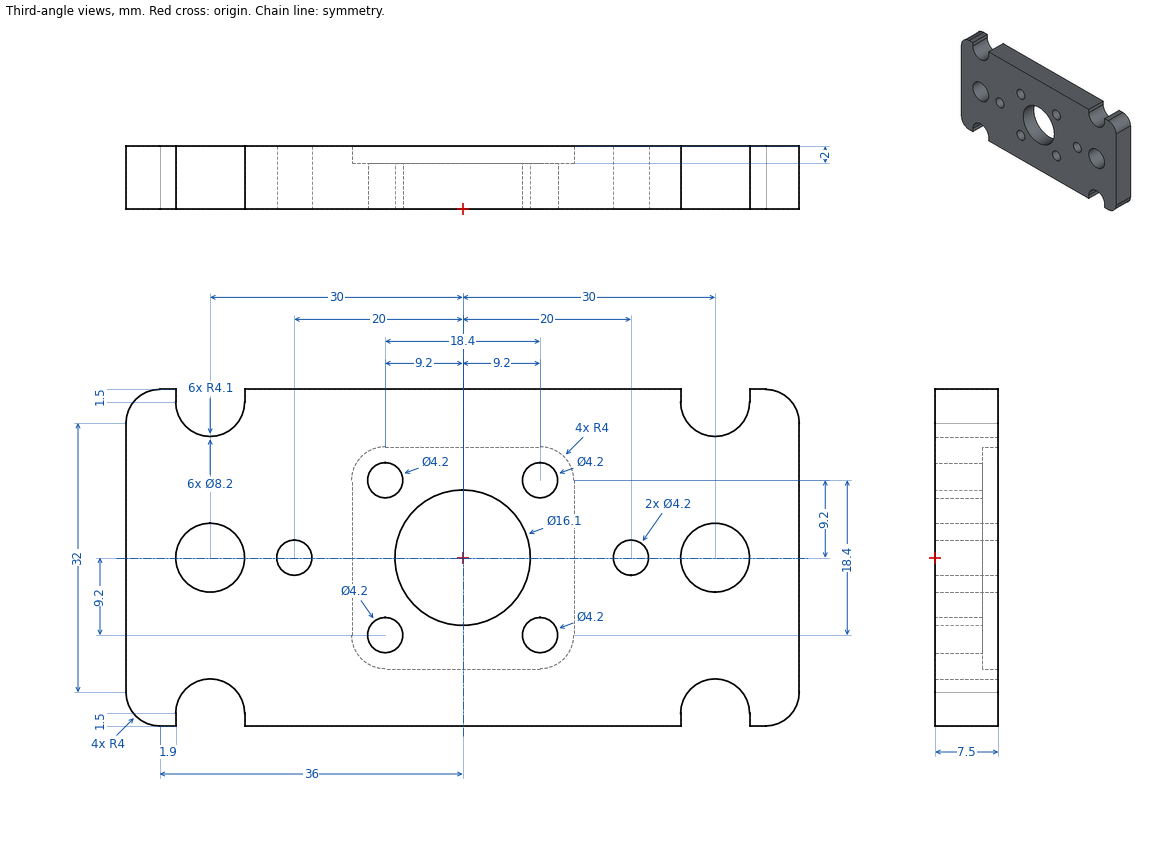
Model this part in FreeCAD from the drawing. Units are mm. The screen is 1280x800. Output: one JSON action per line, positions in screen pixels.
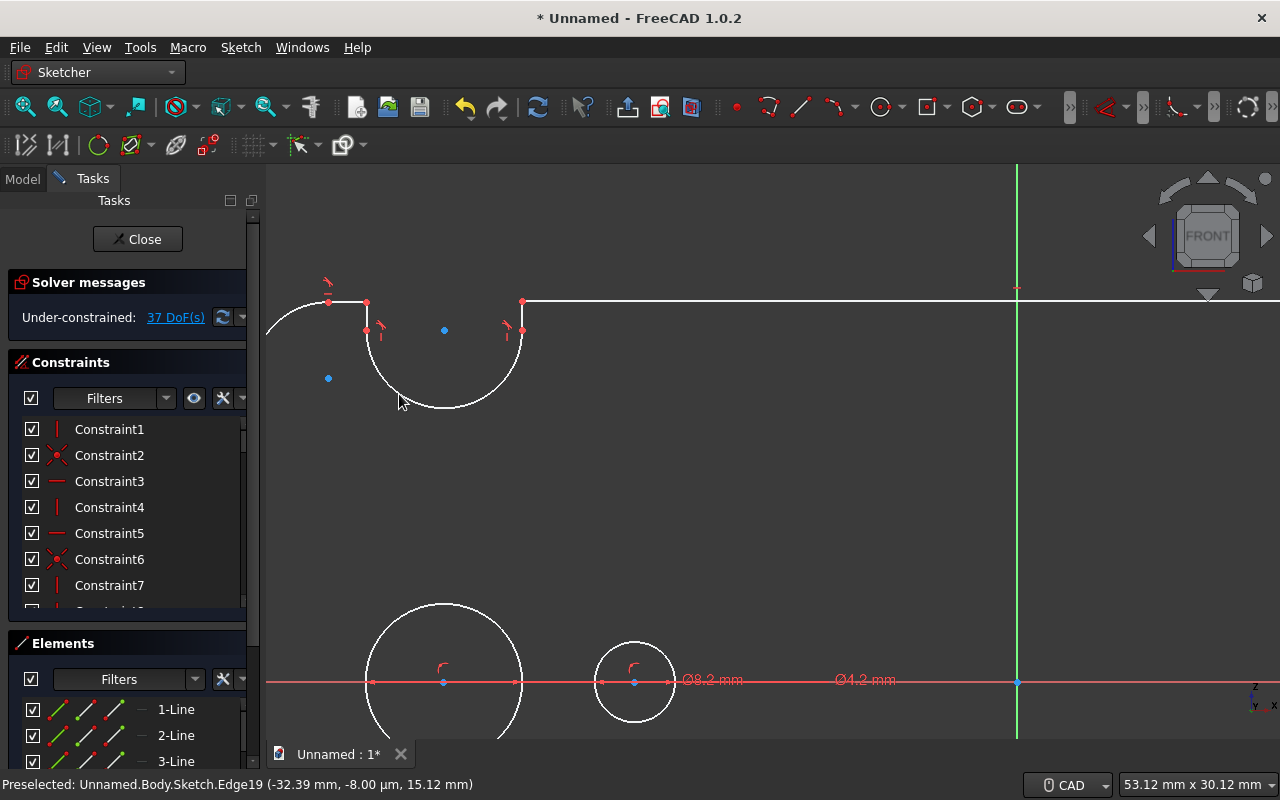
{"action": "scroll", "coordinate": [523, 317], "scroll_direction": "down", "scroll_amount": 5}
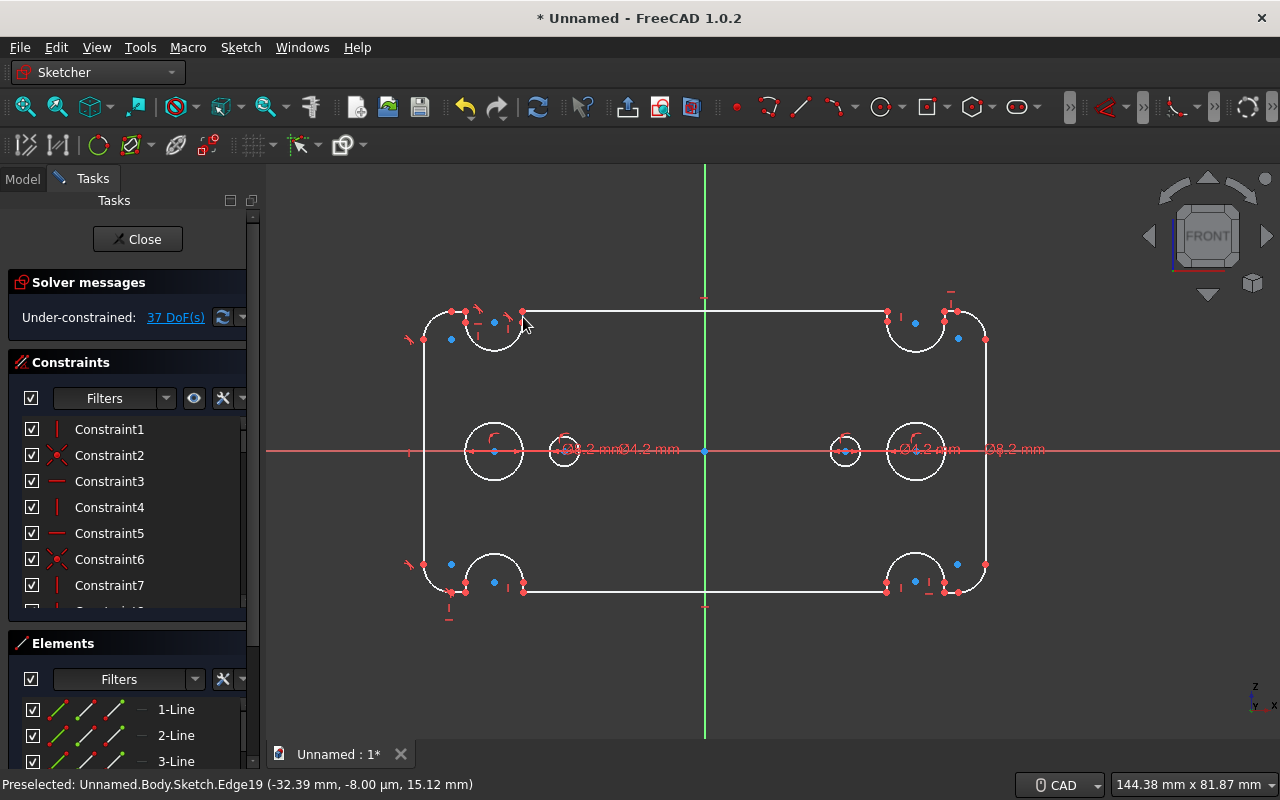
{"action": "scroll", "coordinate": [887, 316], "scroll_direction": "up", "scroll_amount": 6}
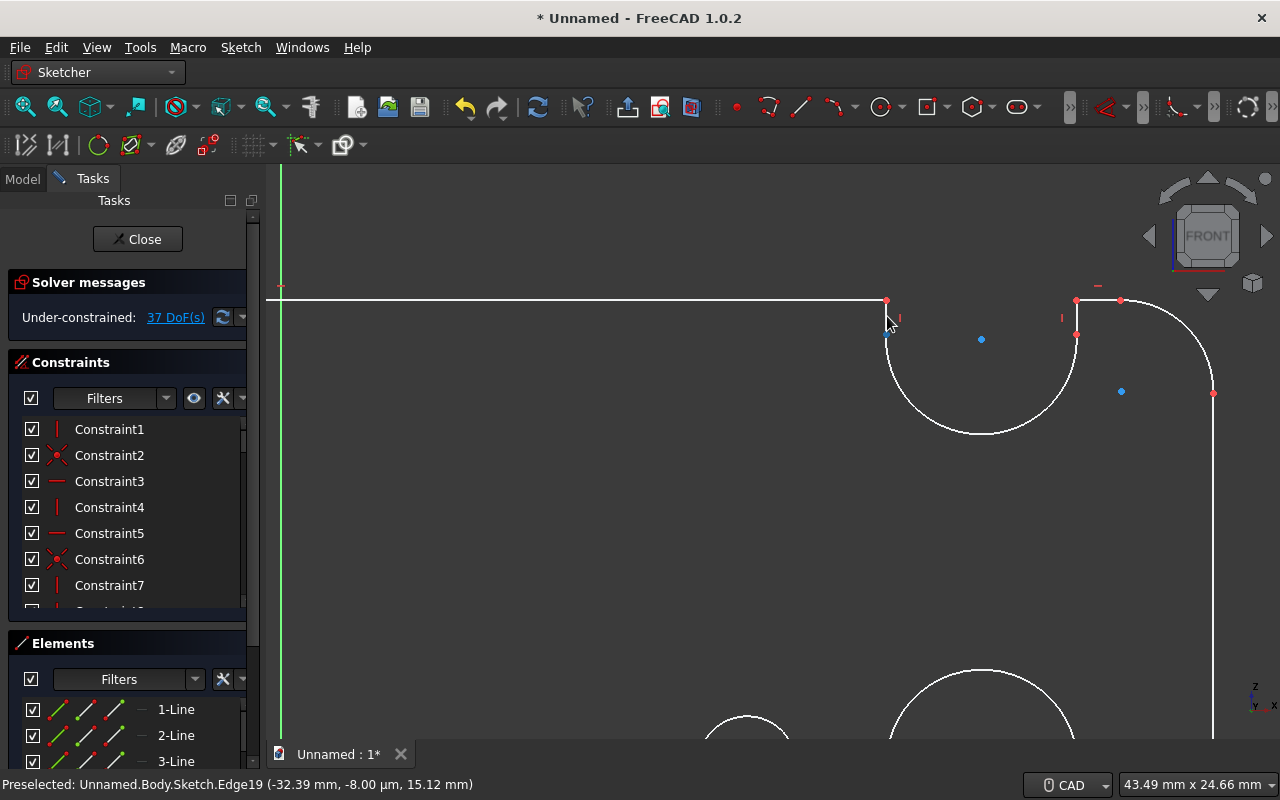
{"action": "left_click", "coordinate": [886, 314]}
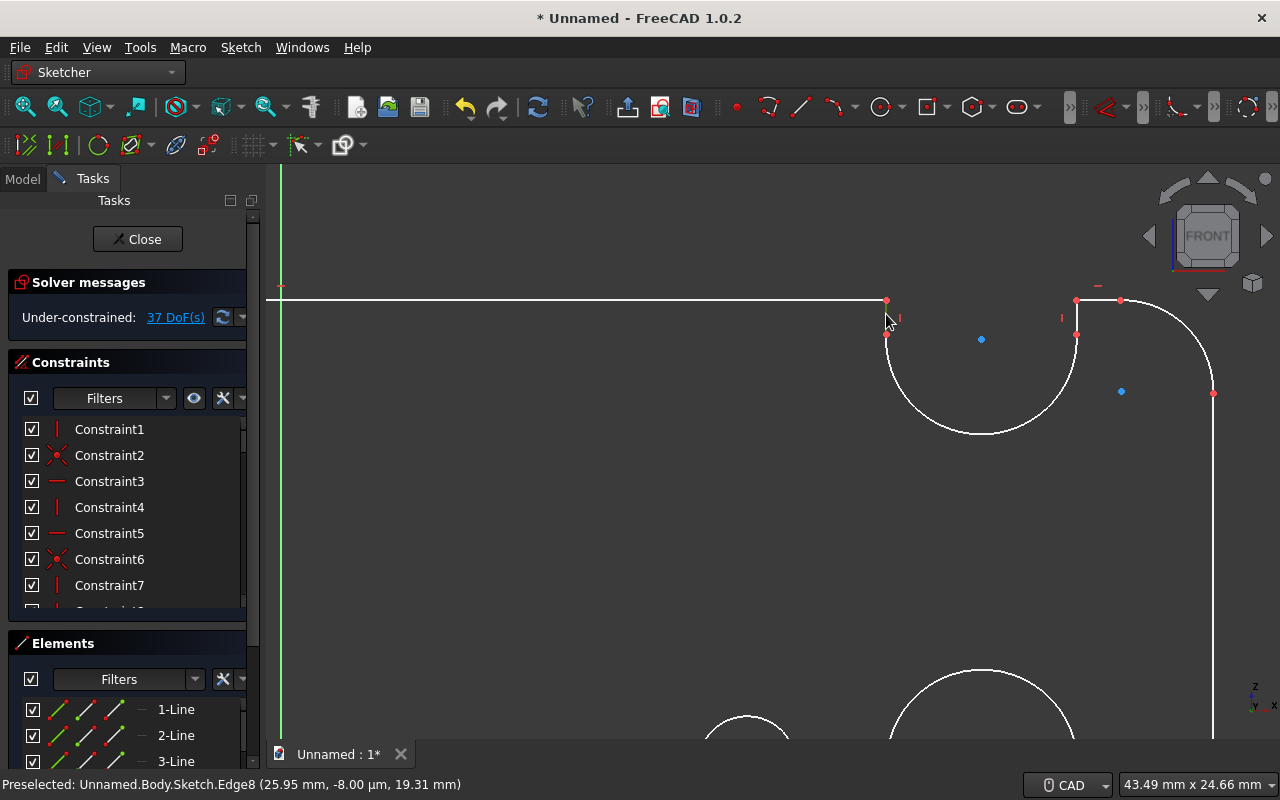
{"action": "scroll", "coordinate": [887, 316], "scroll_direction": "down", "scroll_amount": 6}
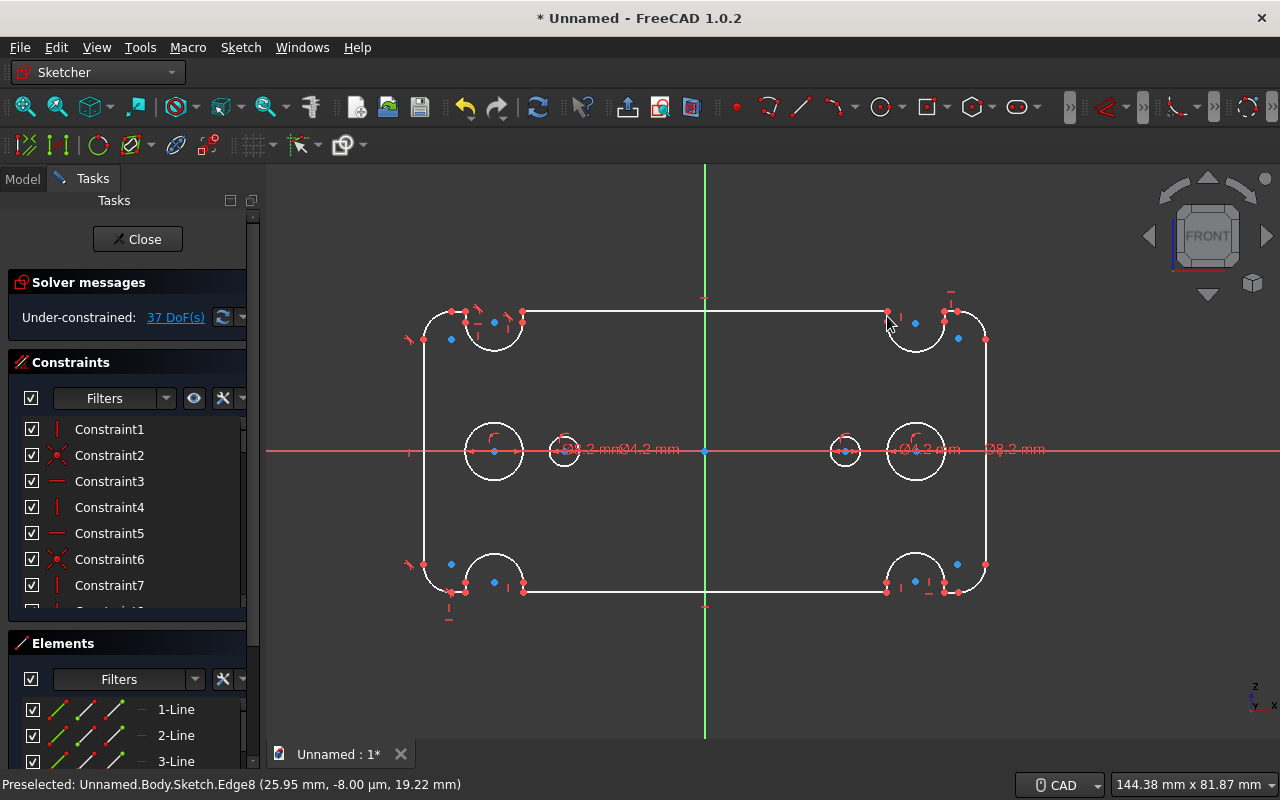
{"action": "left_click", "coordinate": [899, 346]}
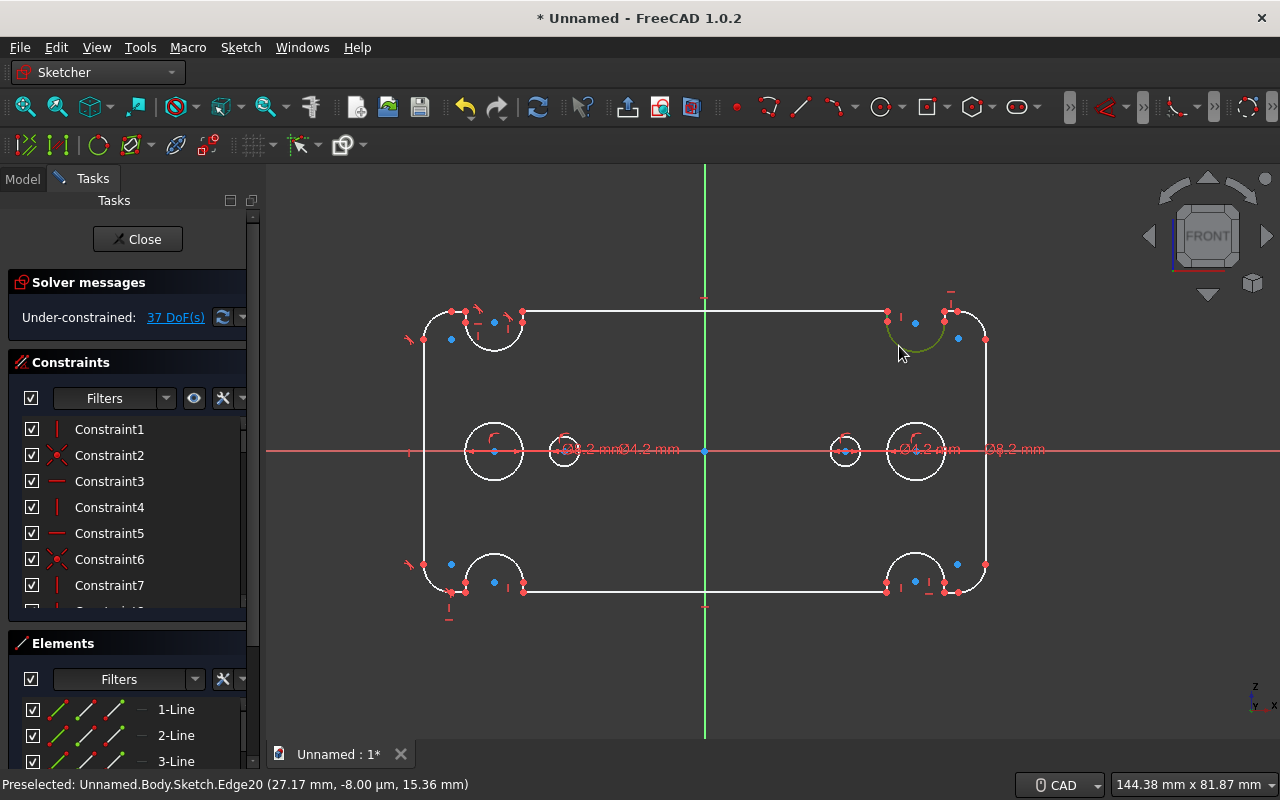
{"action": "key", "text": "t"}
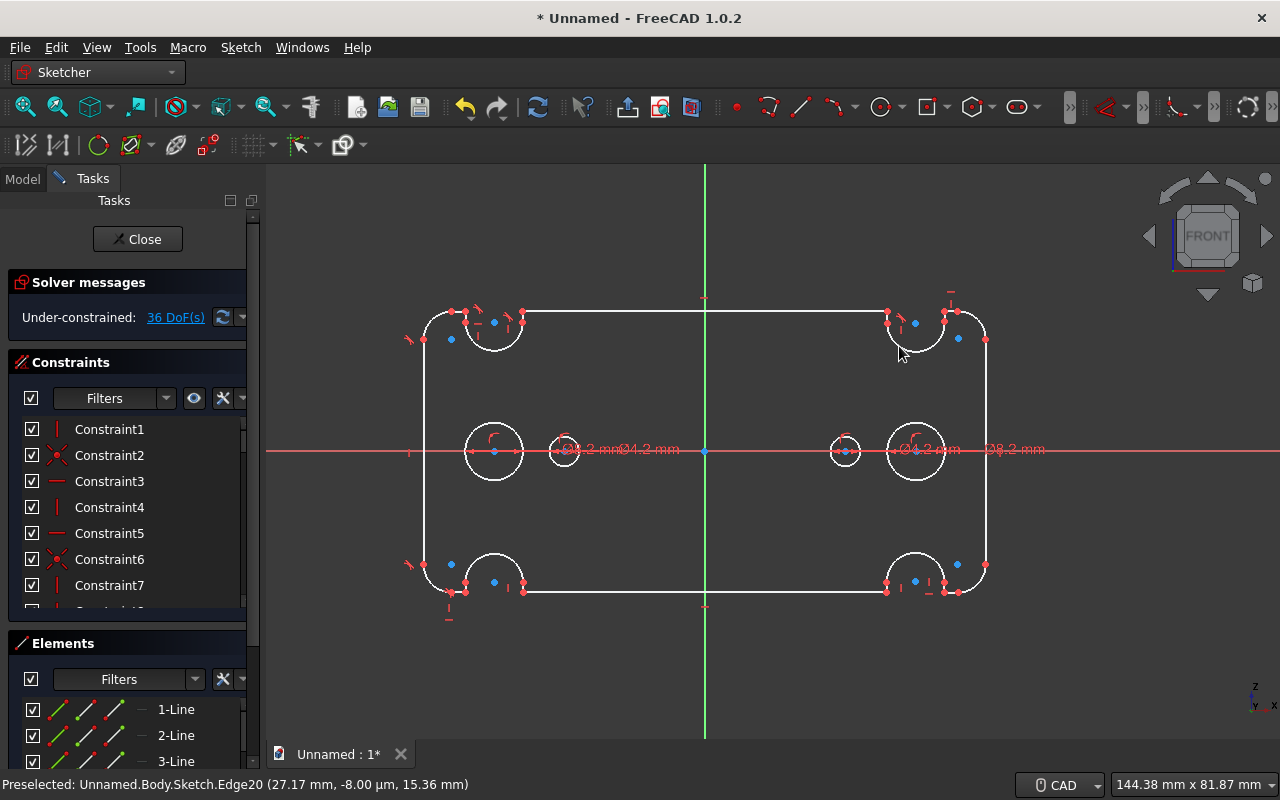
{"action": "scroll", "coordinate": [945, 317], "scroll_direction": "up", "scroll_amount": 5}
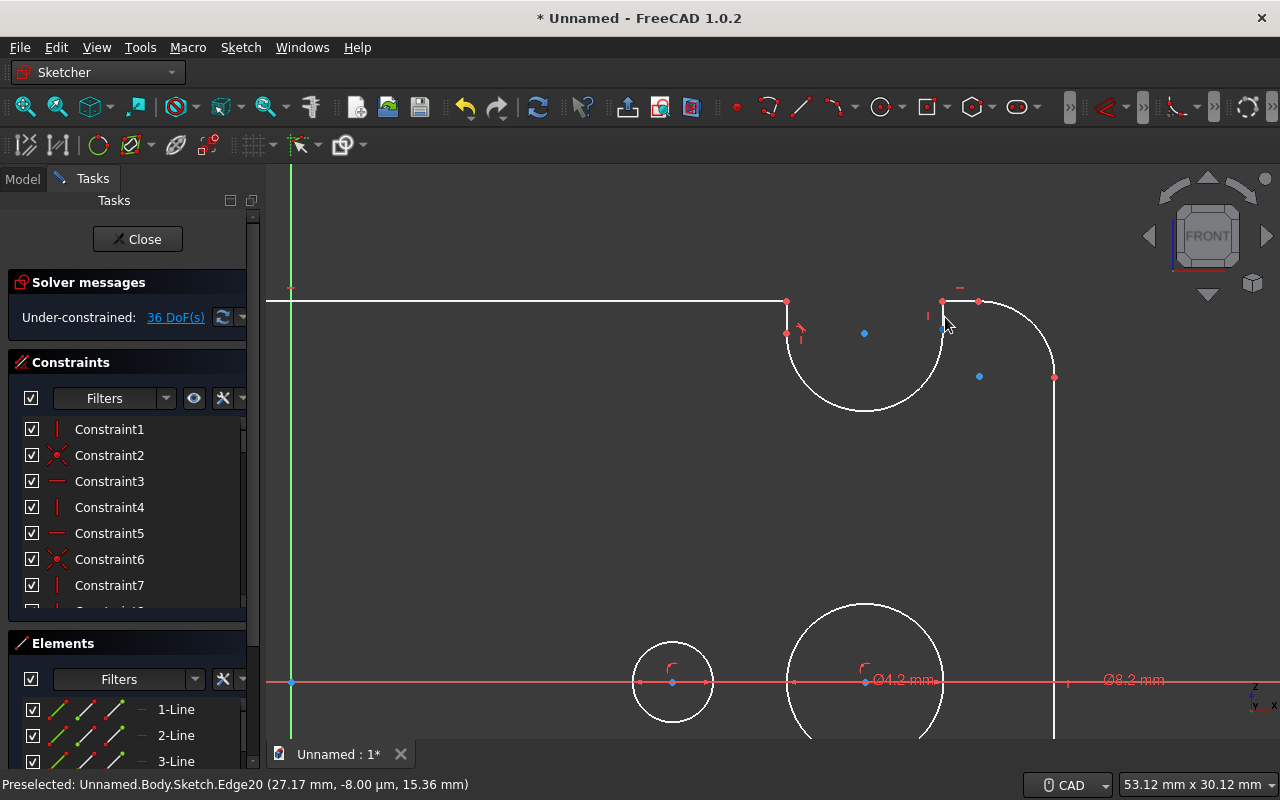
{"action": "left_click", "coordinate": [943, 316]}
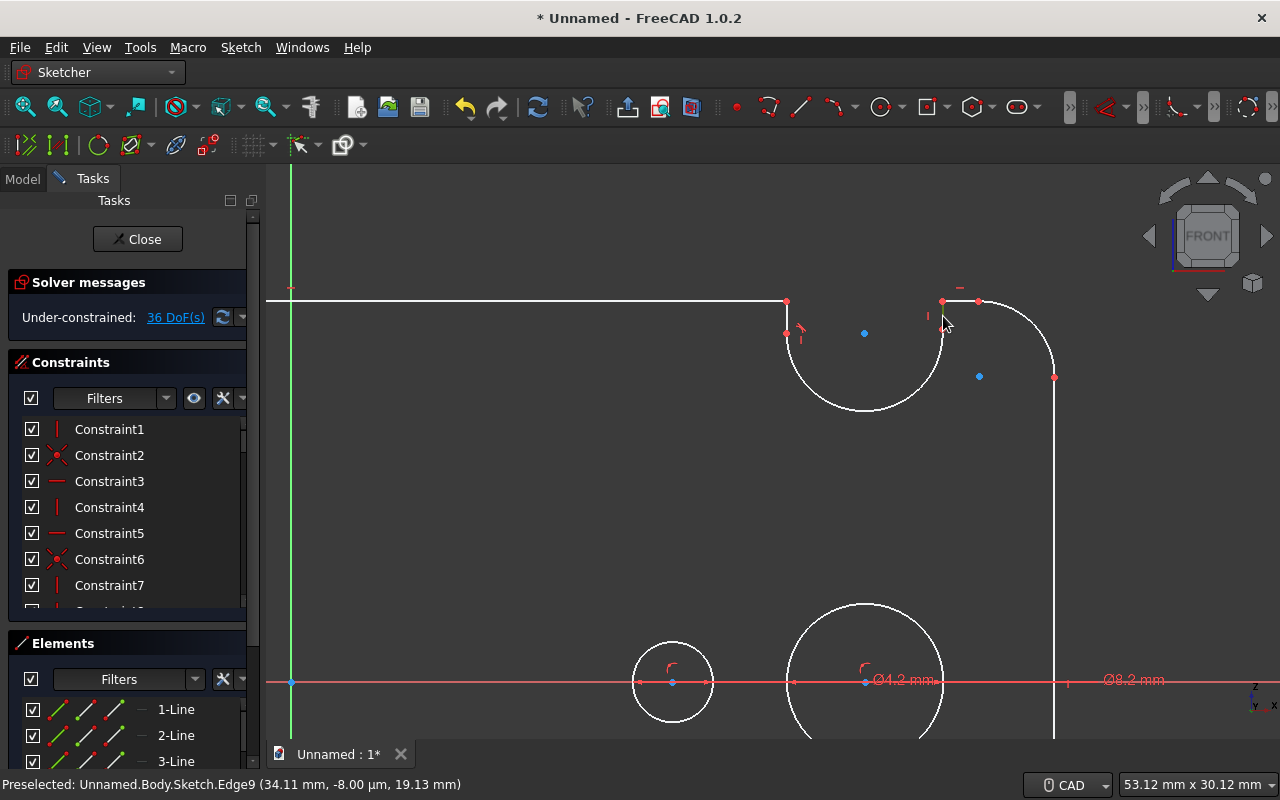
{"action": "left_click", "coordinate": [820, 397]}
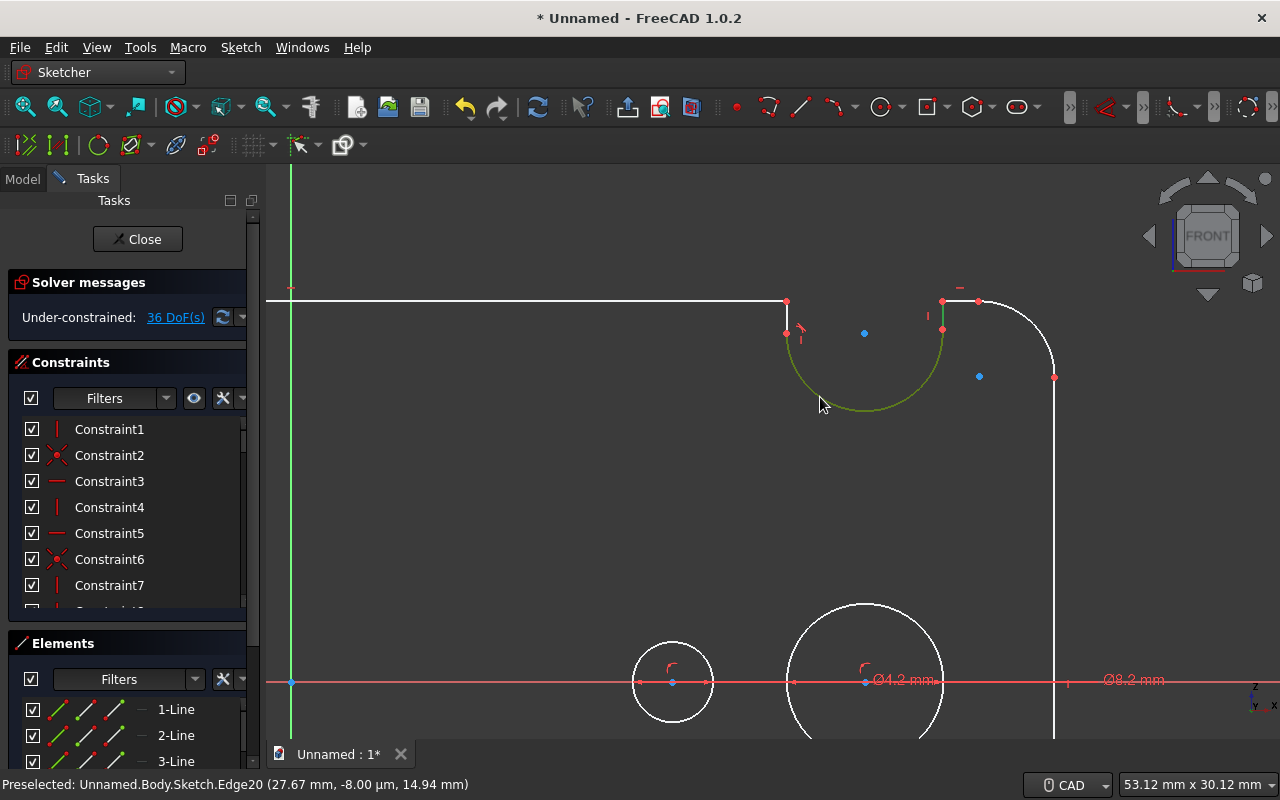
{"action": "key", "text": "t"}